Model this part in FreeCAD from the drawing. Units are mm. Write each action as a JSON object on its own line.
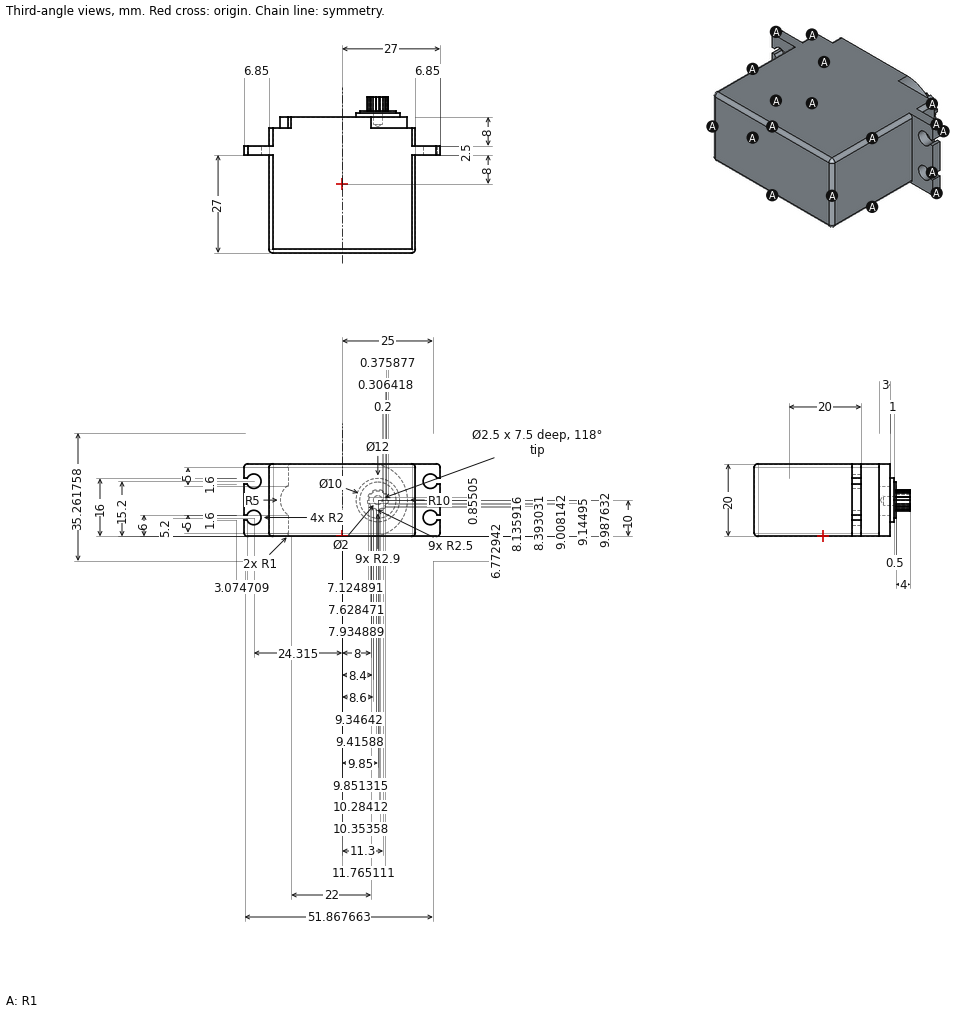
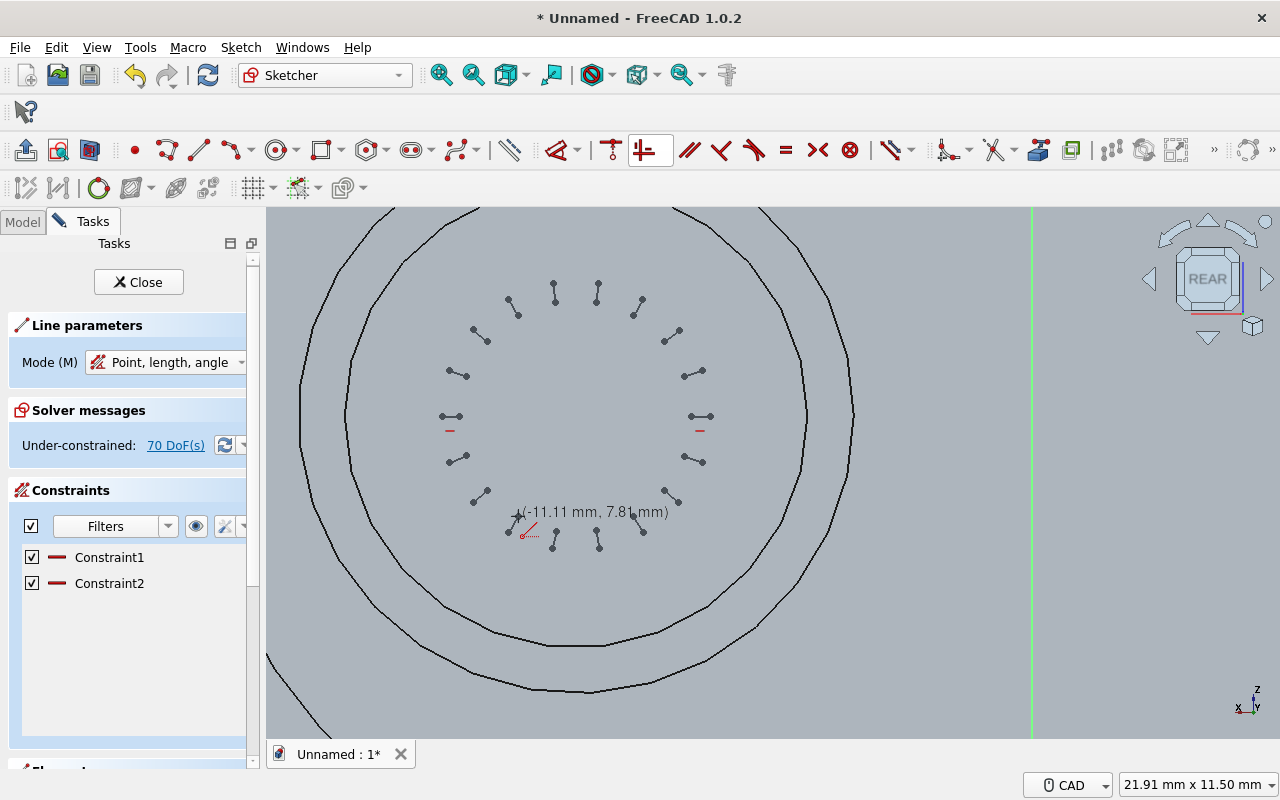
{"action": "left_click", "coordinate": [232, 150]}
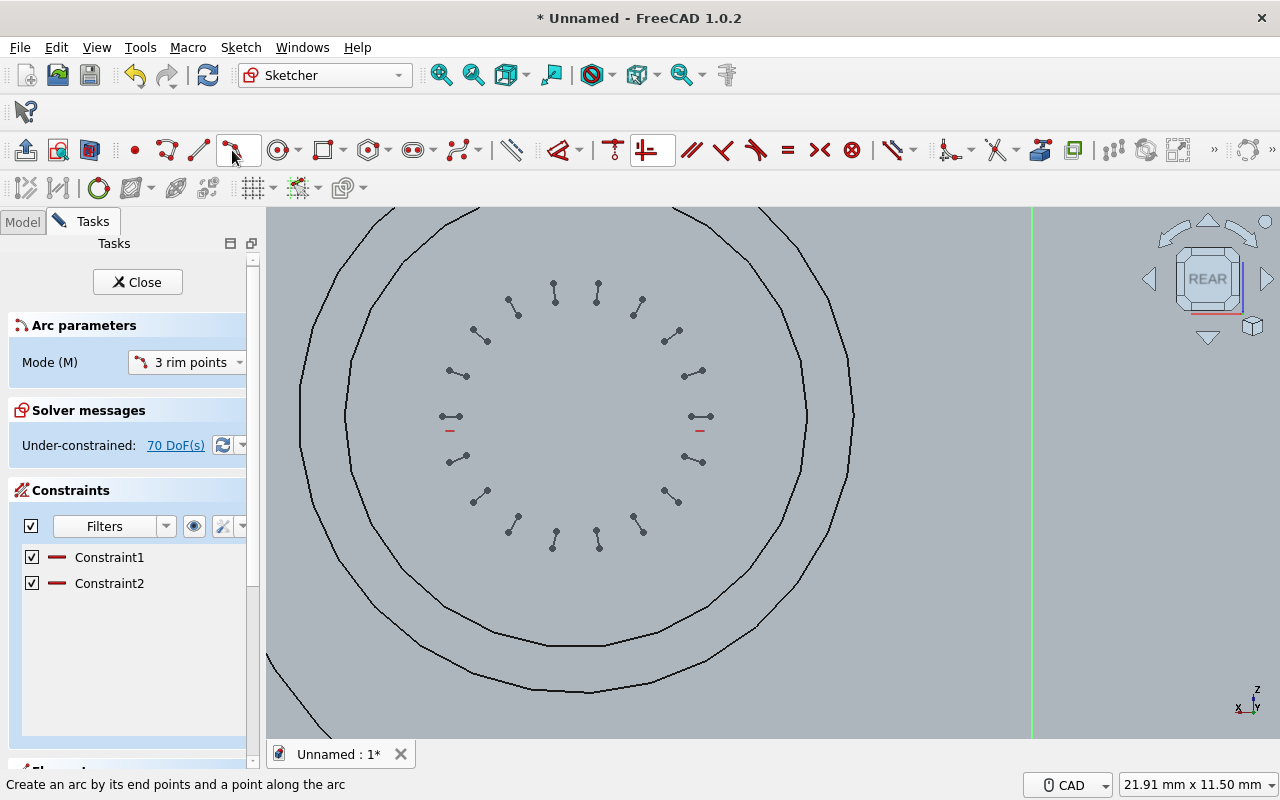
{"action": "scroll", "coordinate": [553, 548], "scroll_direction": "up", "scroll_amount": 3}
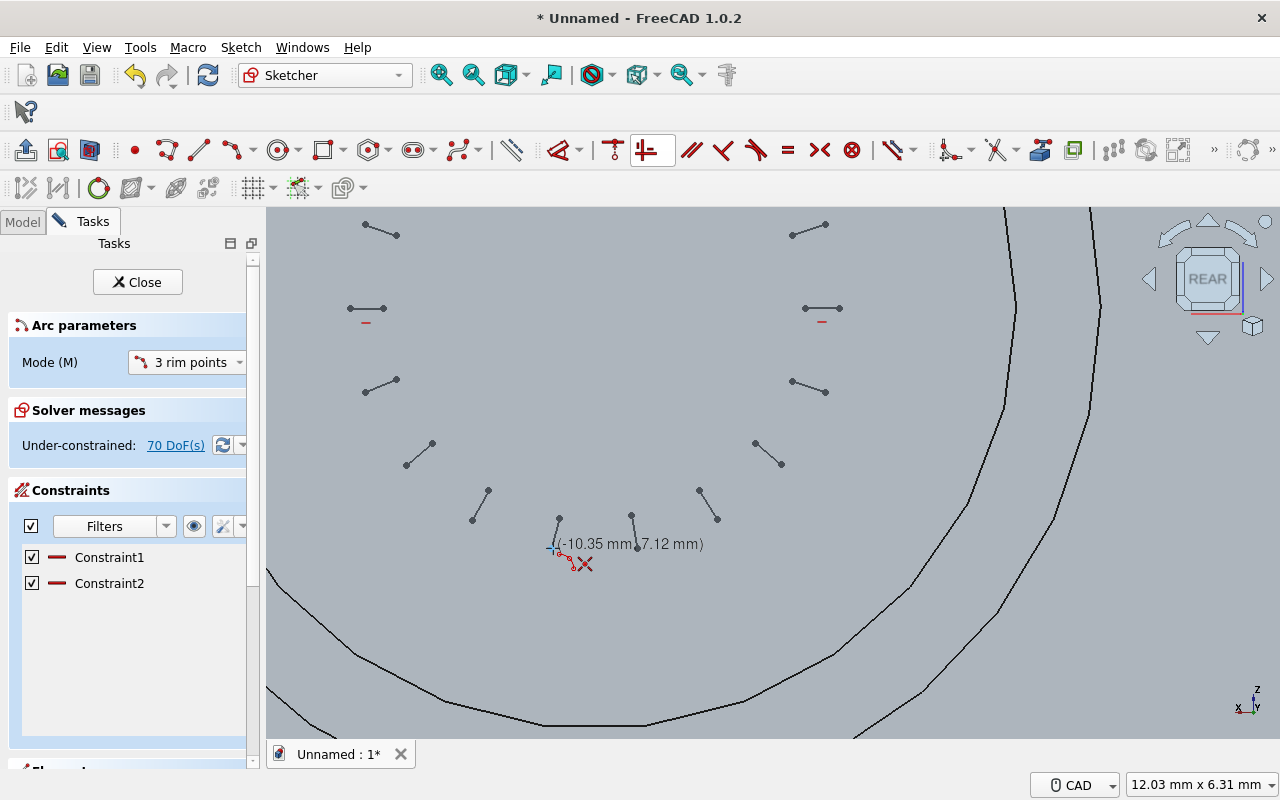
{"action": "left_click", "coordinate": [552, 549]}
{"action": "left_click", "coordinate": [637, 549]}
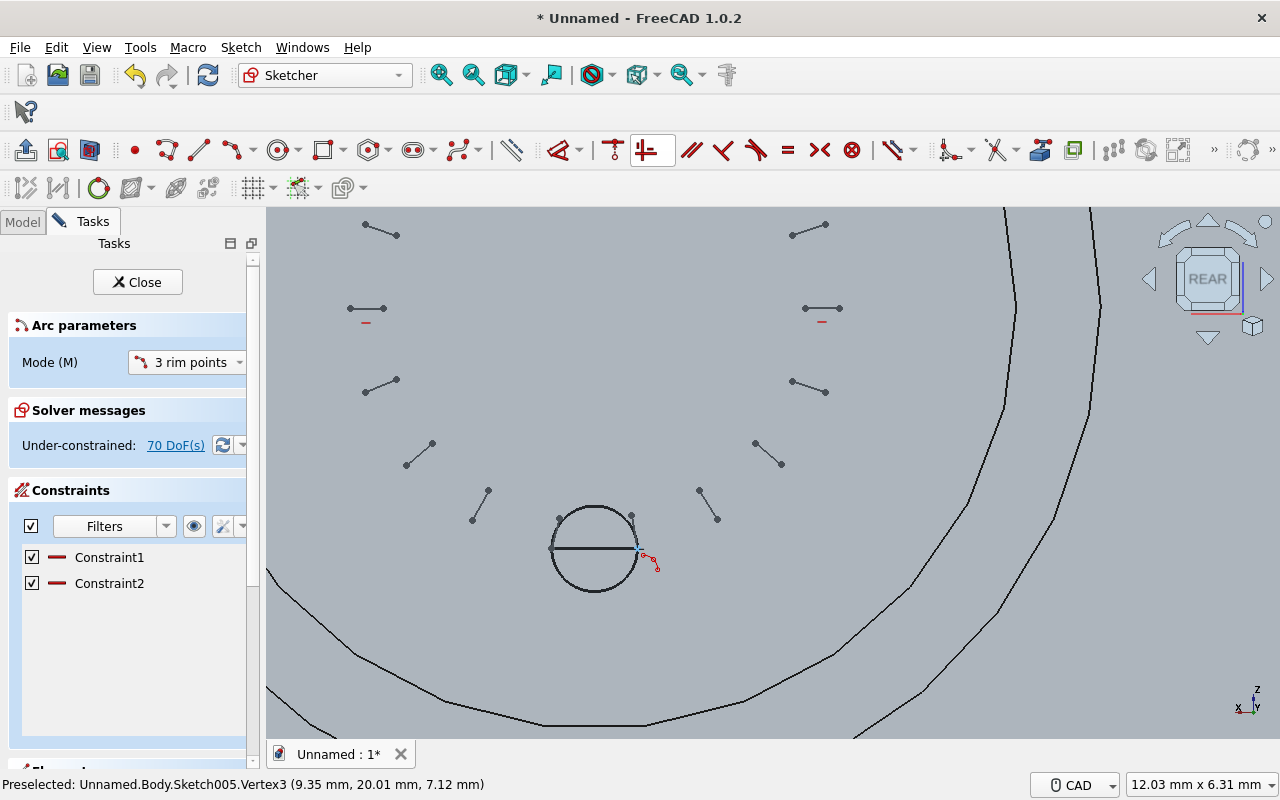
{"action": "scroll", "coordinate": [595, 551], "scroll_direction": "up", "scroll_amount": 8}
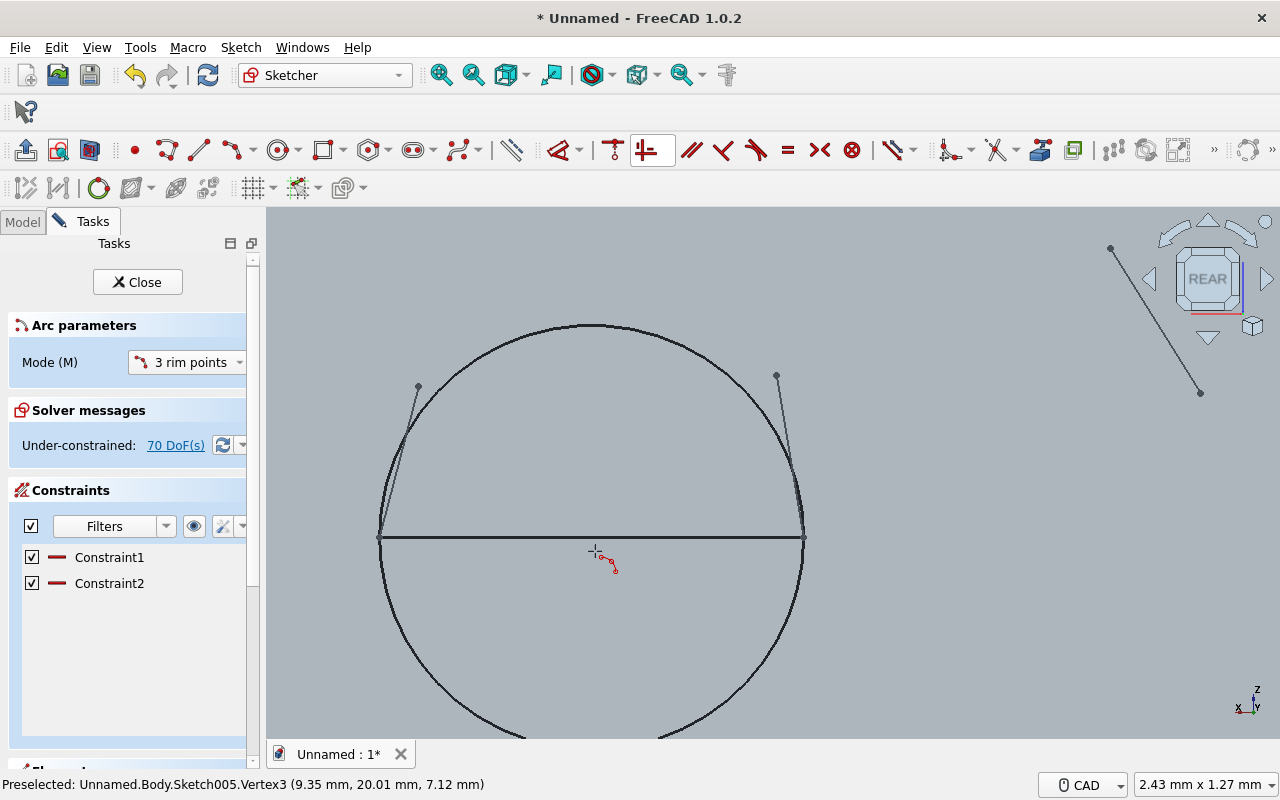
{"action": "left_click", "coordinate": [593, 548]}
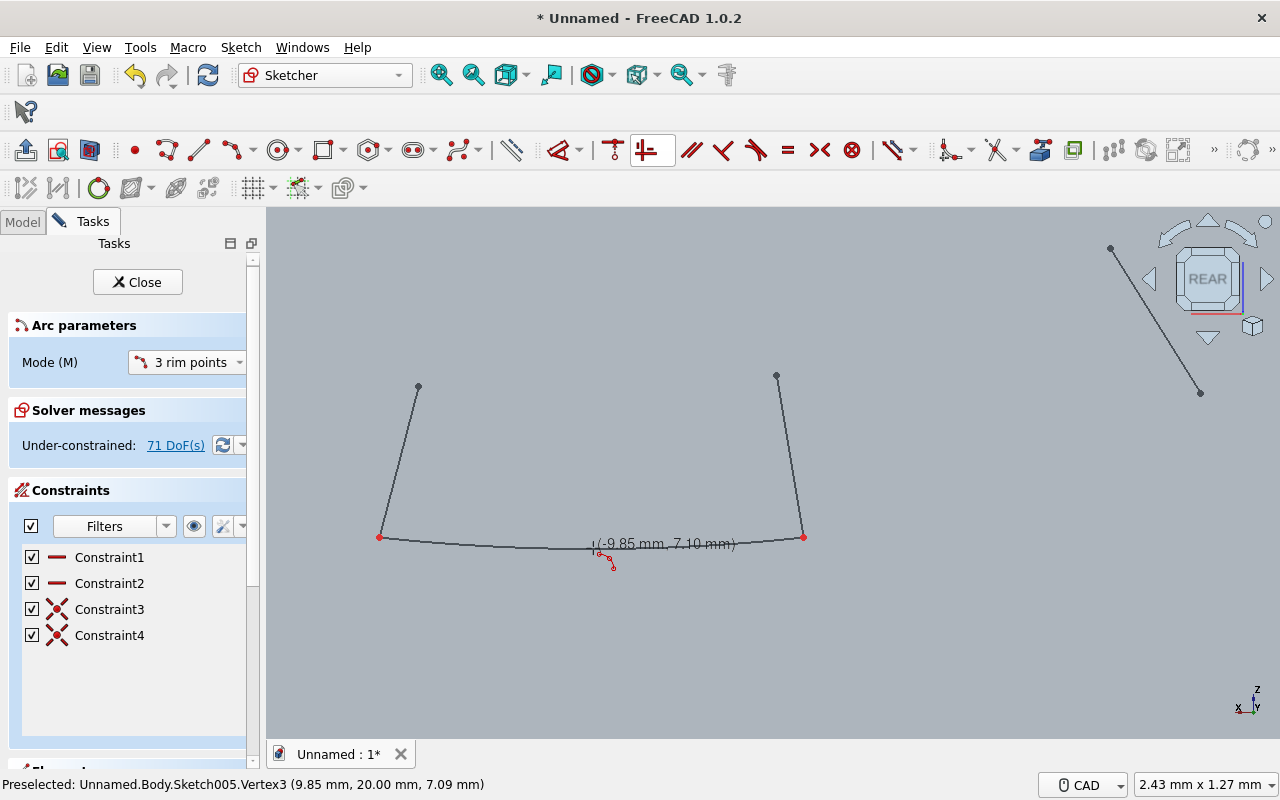
{"action": "scroll", "coordinate": [618, 450], "scroll_direction": "down", "scroll_amount": 14}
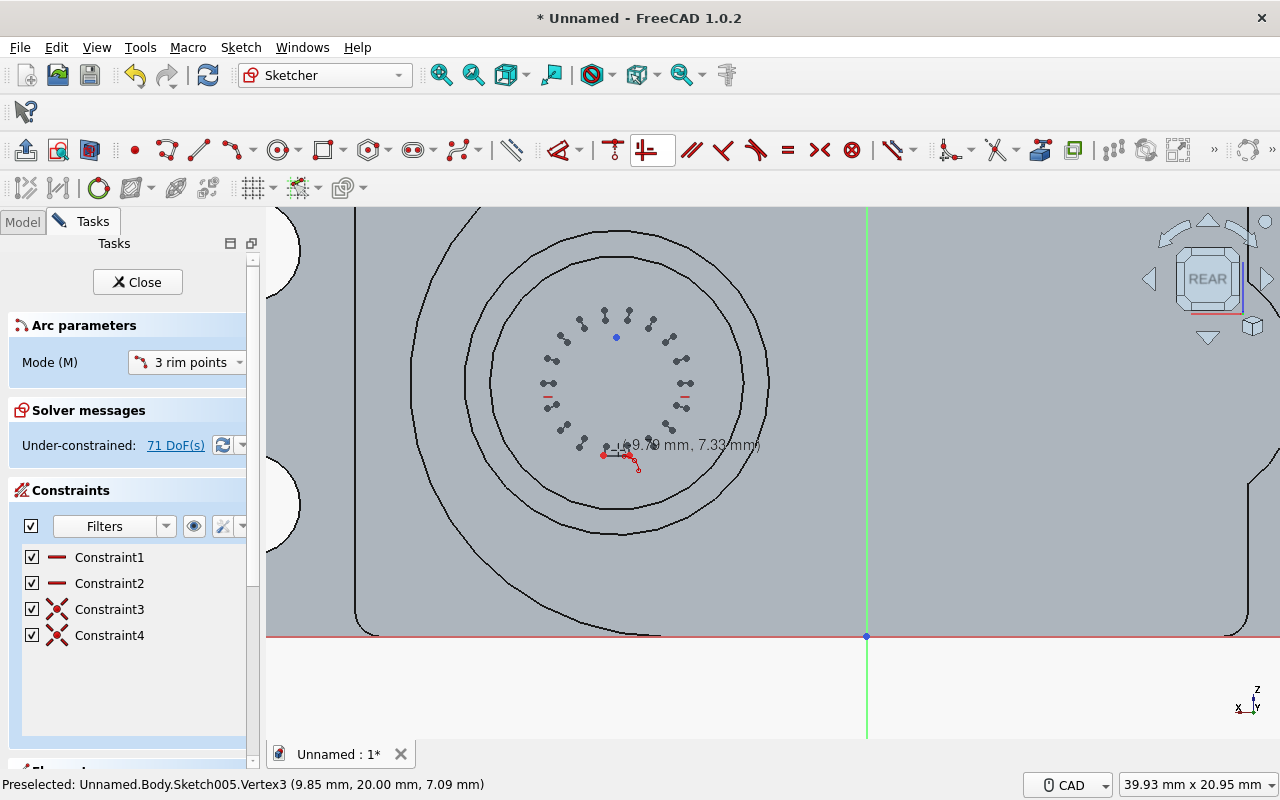
{"action": "scroll", "coordinate": [628, 445], "scroll_direction": "up", "scroll_amount": 6}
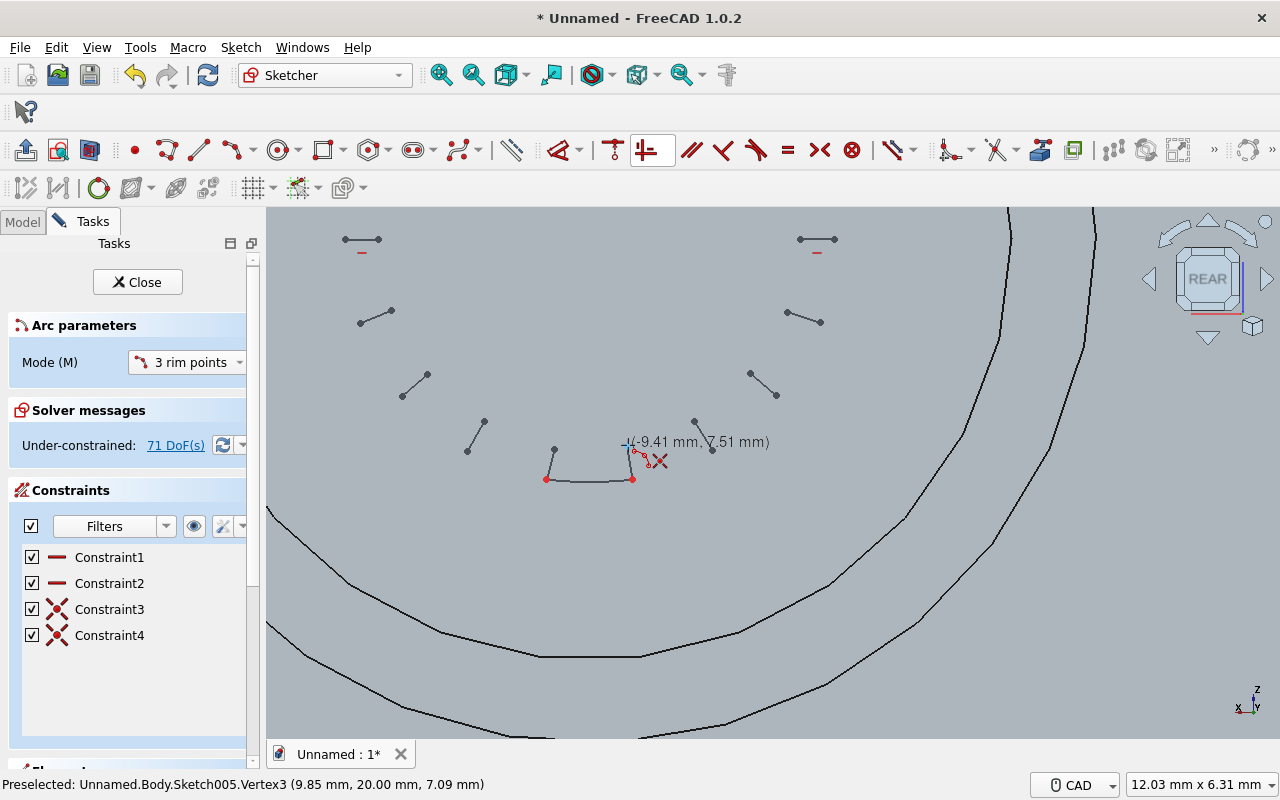
{"action": "left_click", "coordinate": [627, 447]}
{"action": "left_click", "coordinate": [695, 421]}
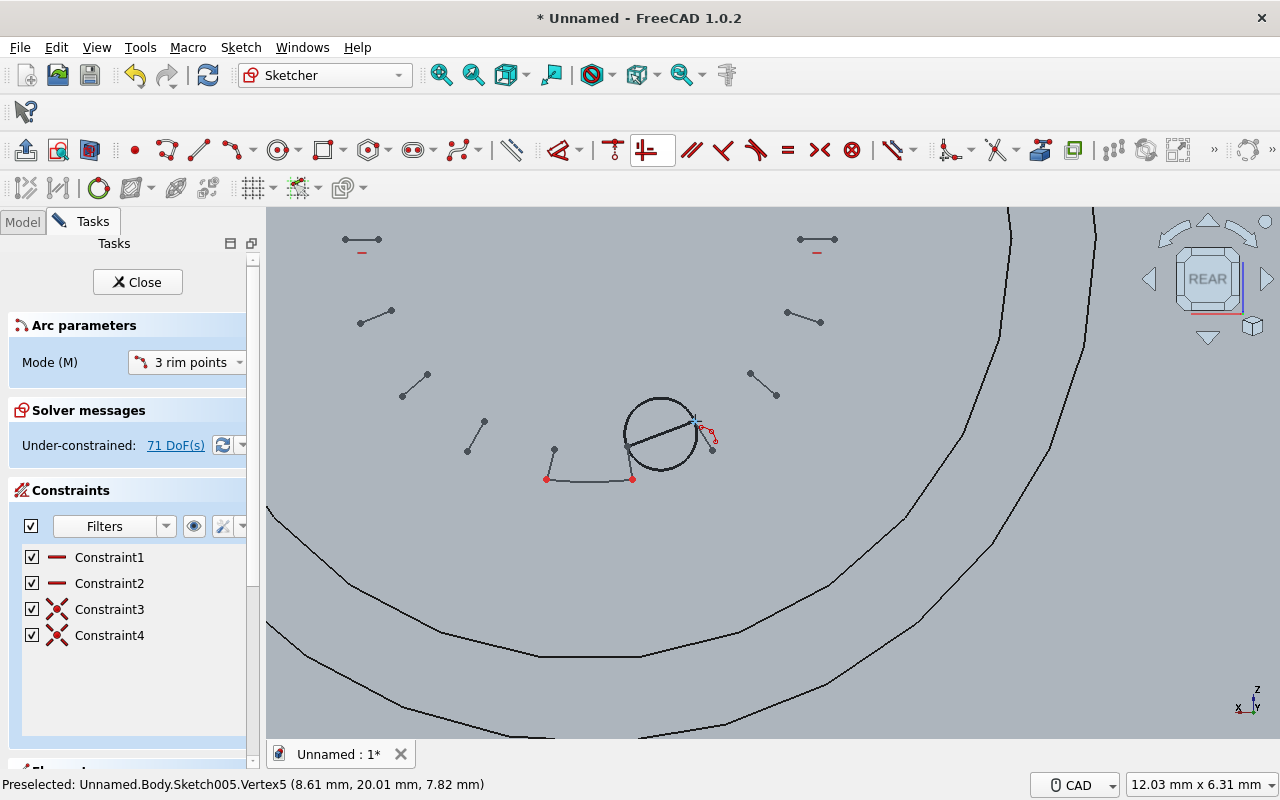
{"action": "scroll", "coordinate": [662, 435], "scroll_direction": "up", "scroll_amount": 9}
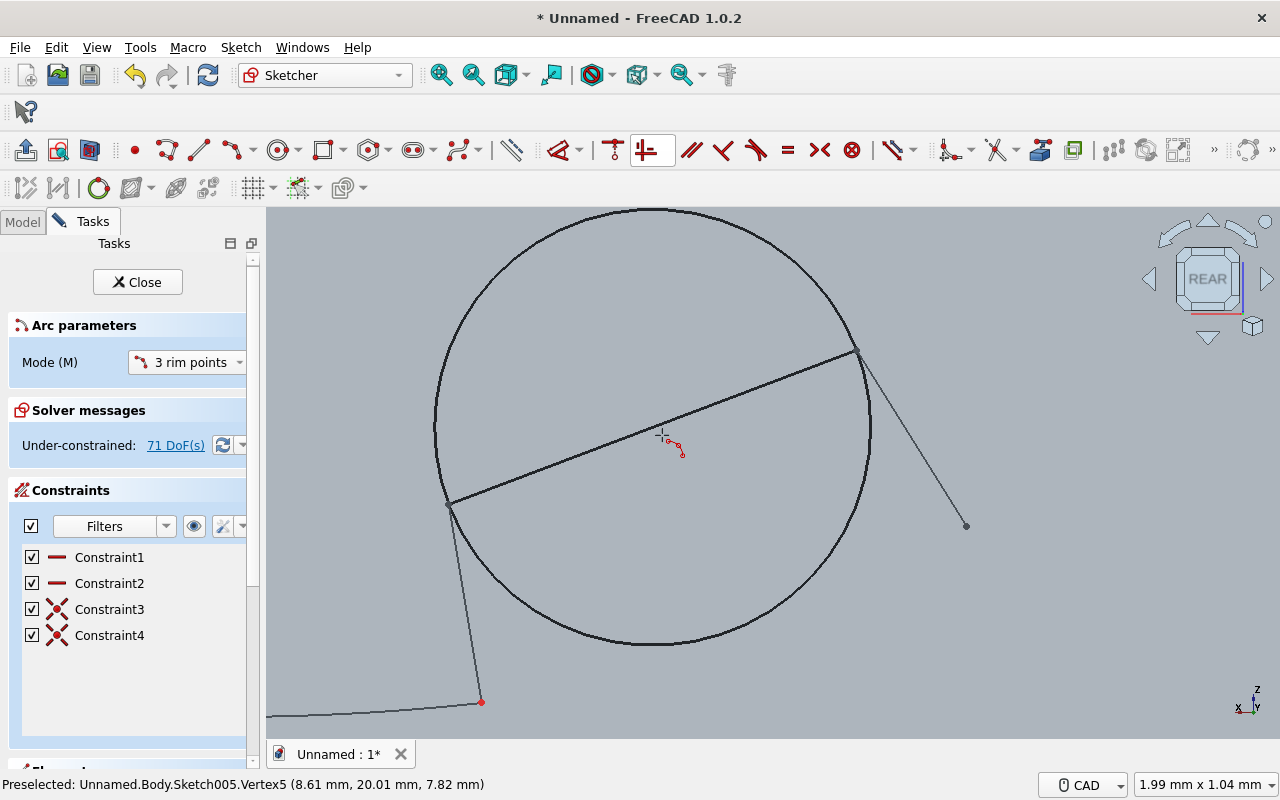
{"action": "left_click", "coordinate": [661, 435]}